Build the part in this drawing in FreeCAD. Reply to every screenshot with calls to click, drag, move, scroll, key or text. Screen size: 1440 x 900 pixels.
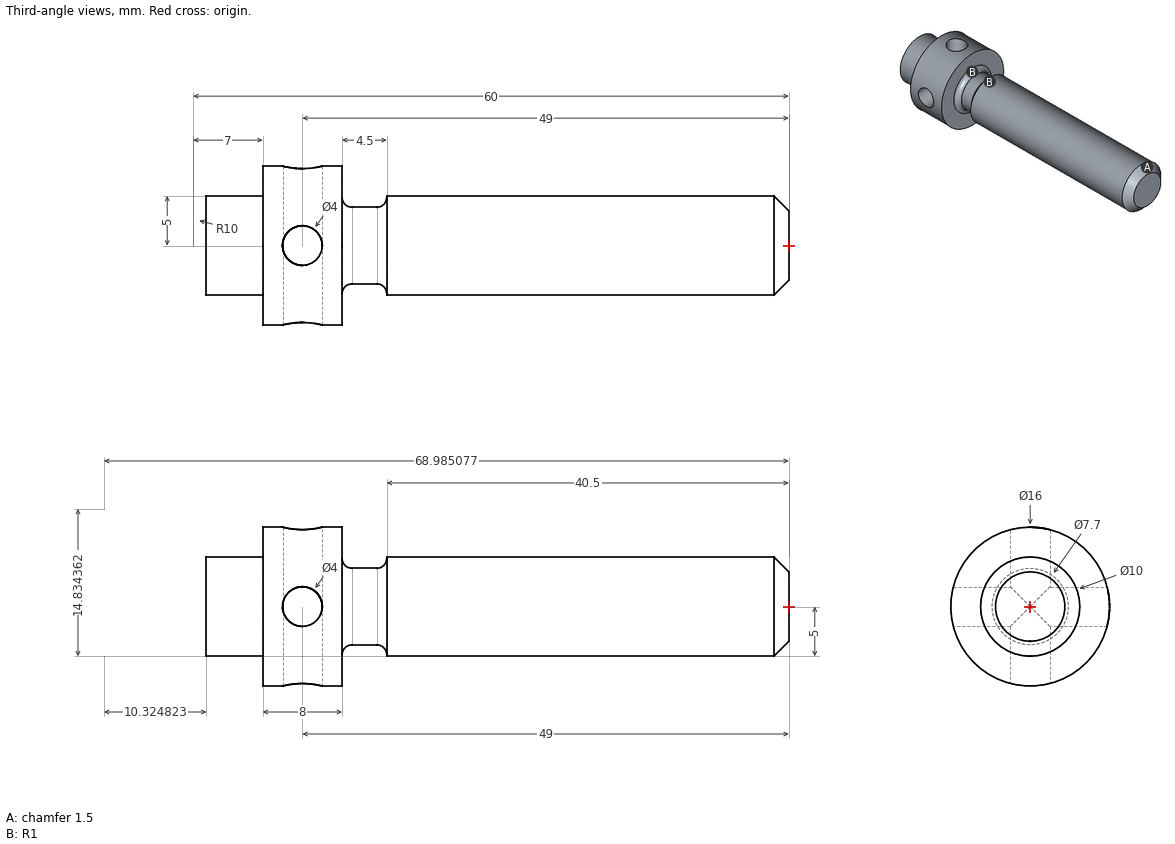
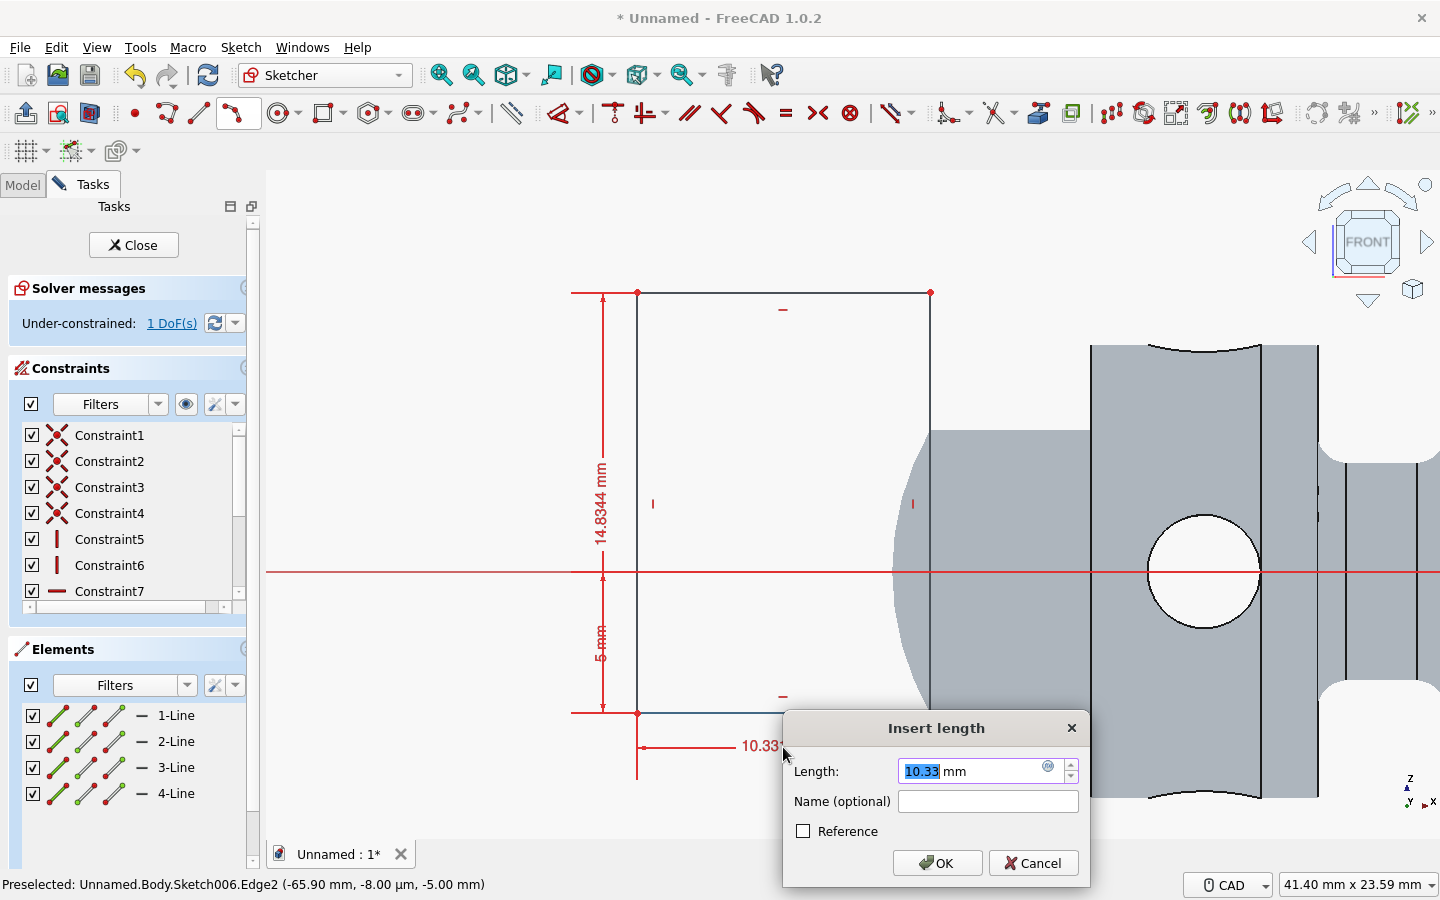
text(10.324823)
key(Return)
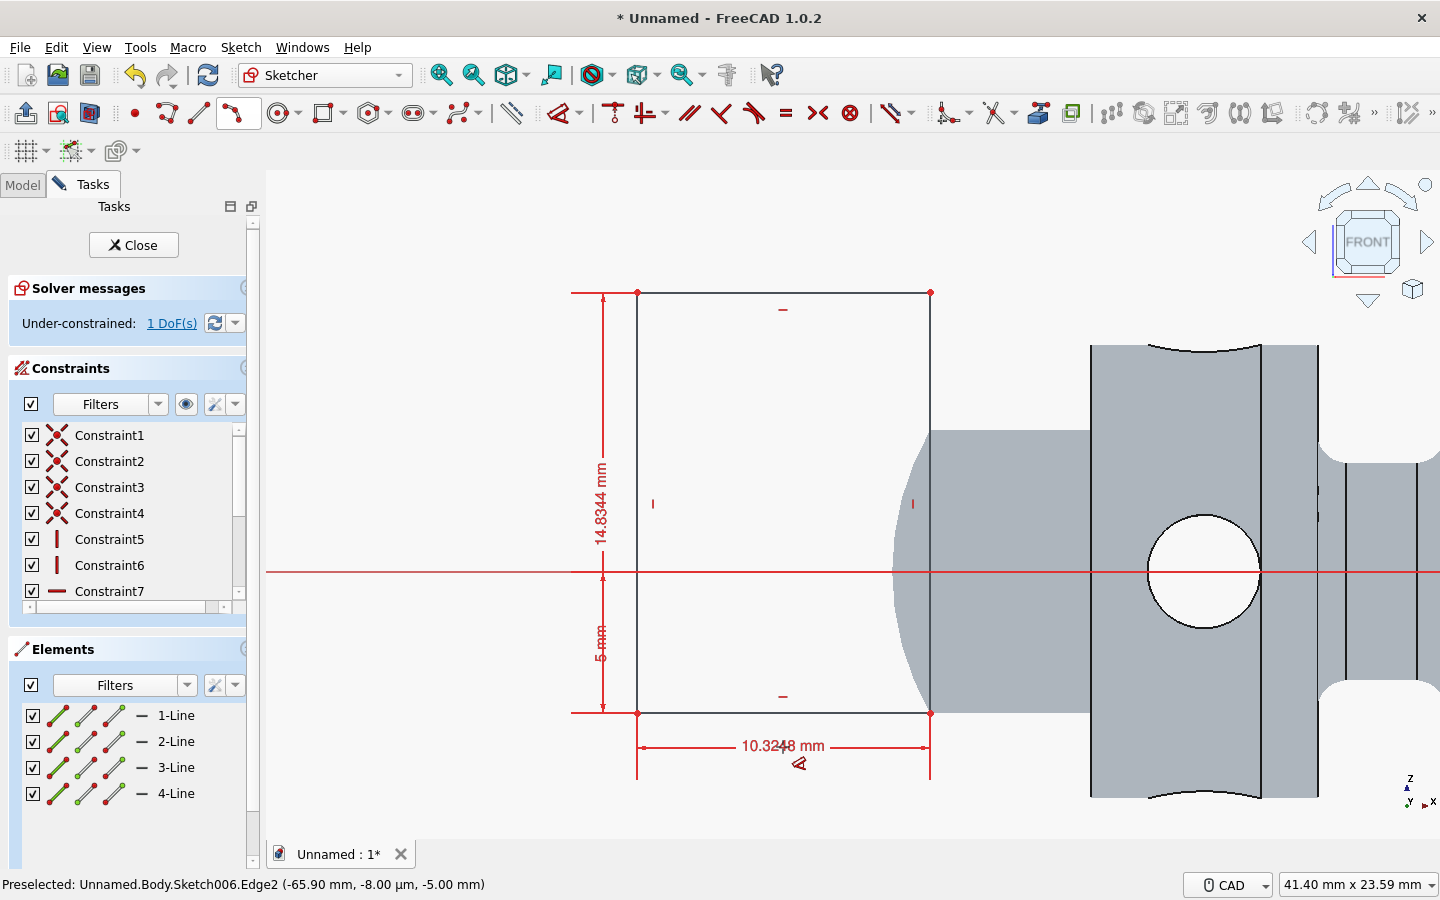
click(637, 293)
click(956, 259)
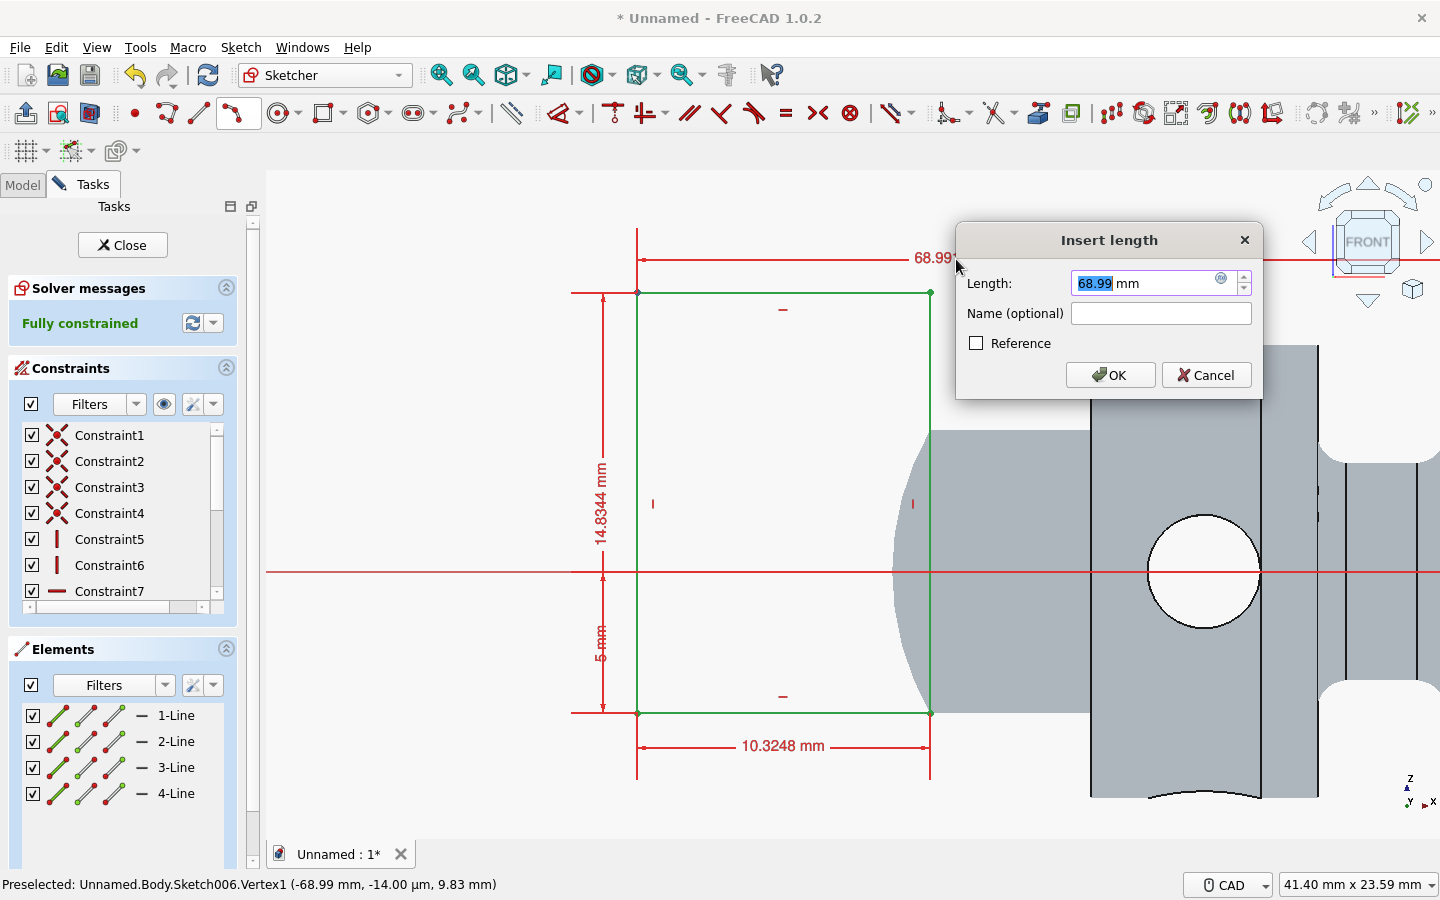
text(68.985077)
key(Return)
key(Escape)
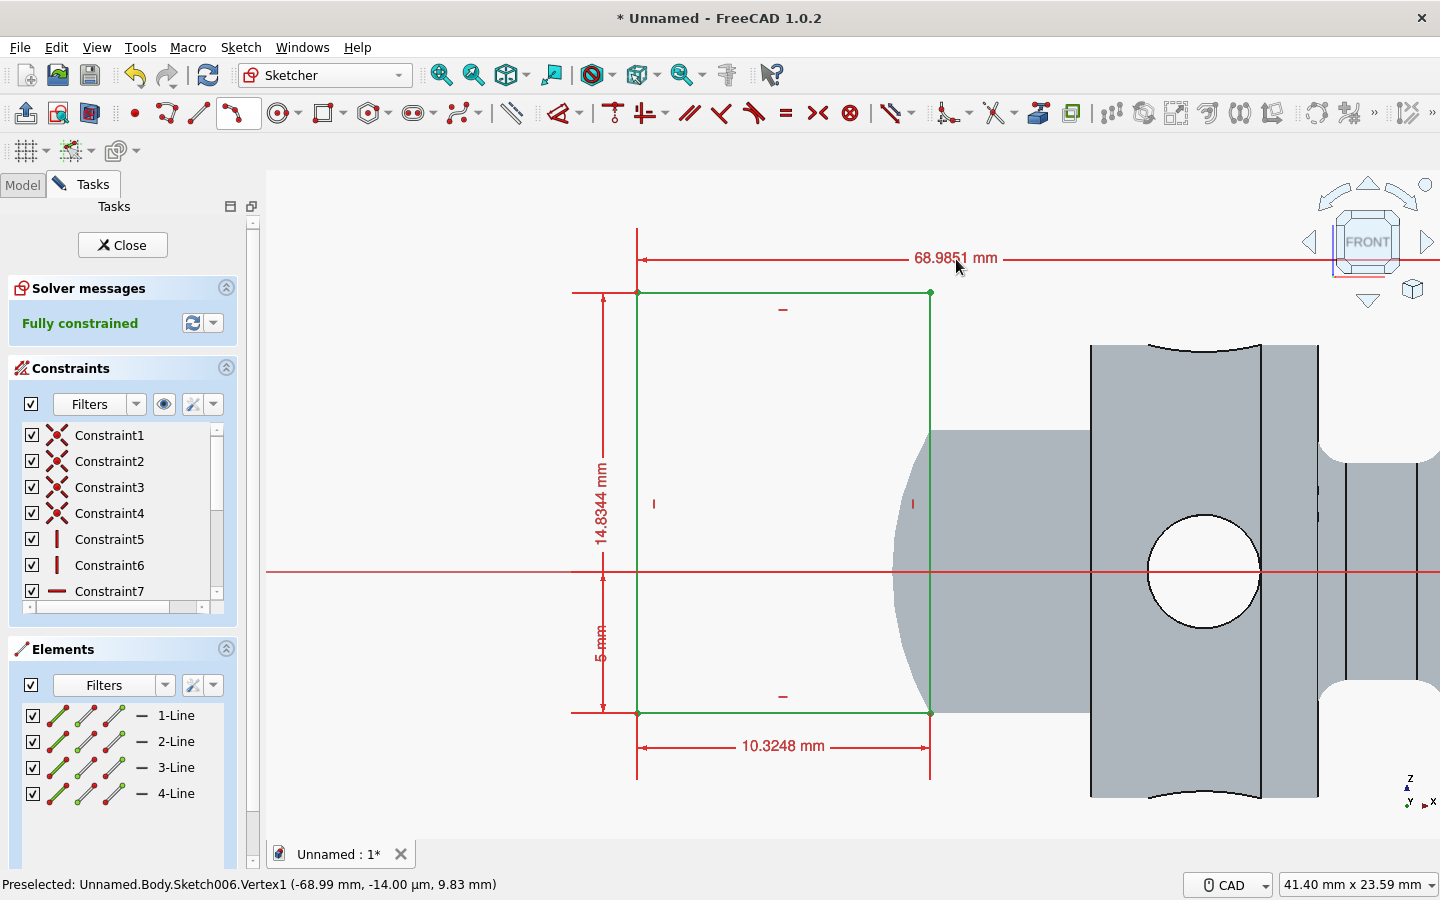
click(123, 245)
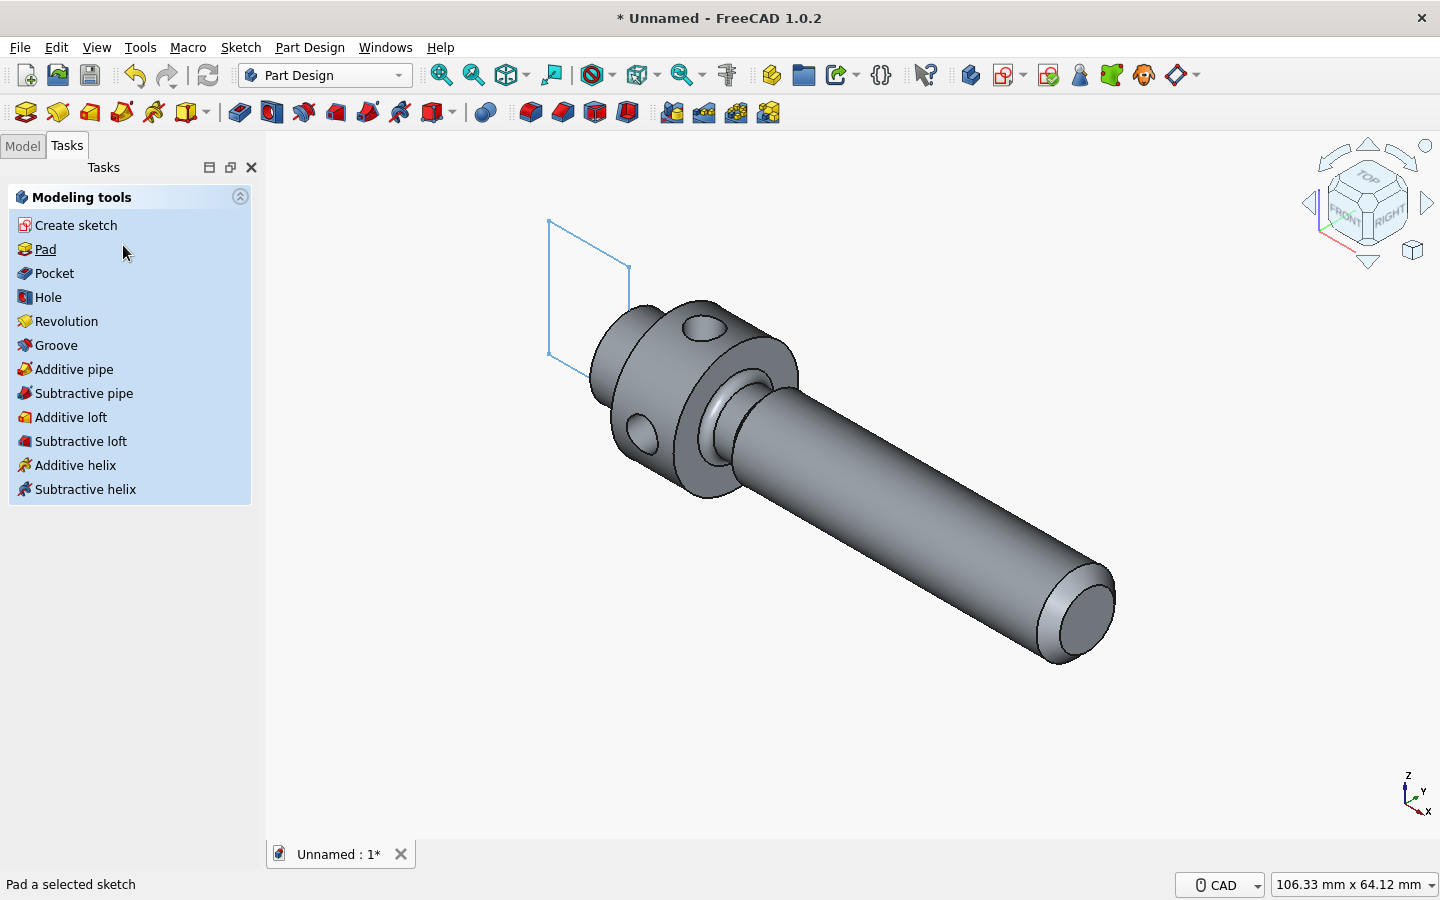
click(240, 112)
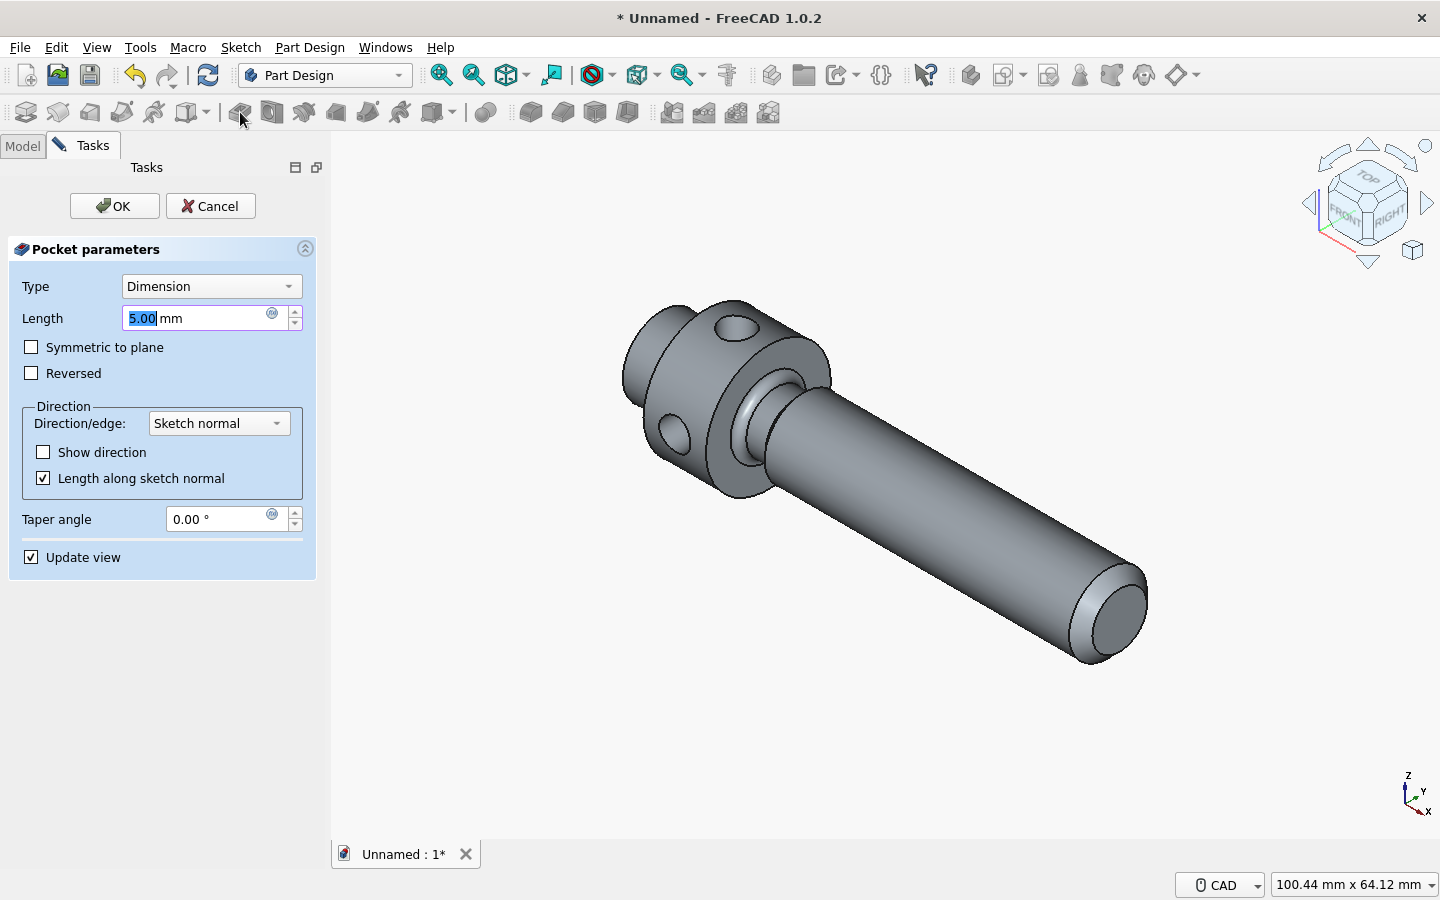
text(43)
key(Tab)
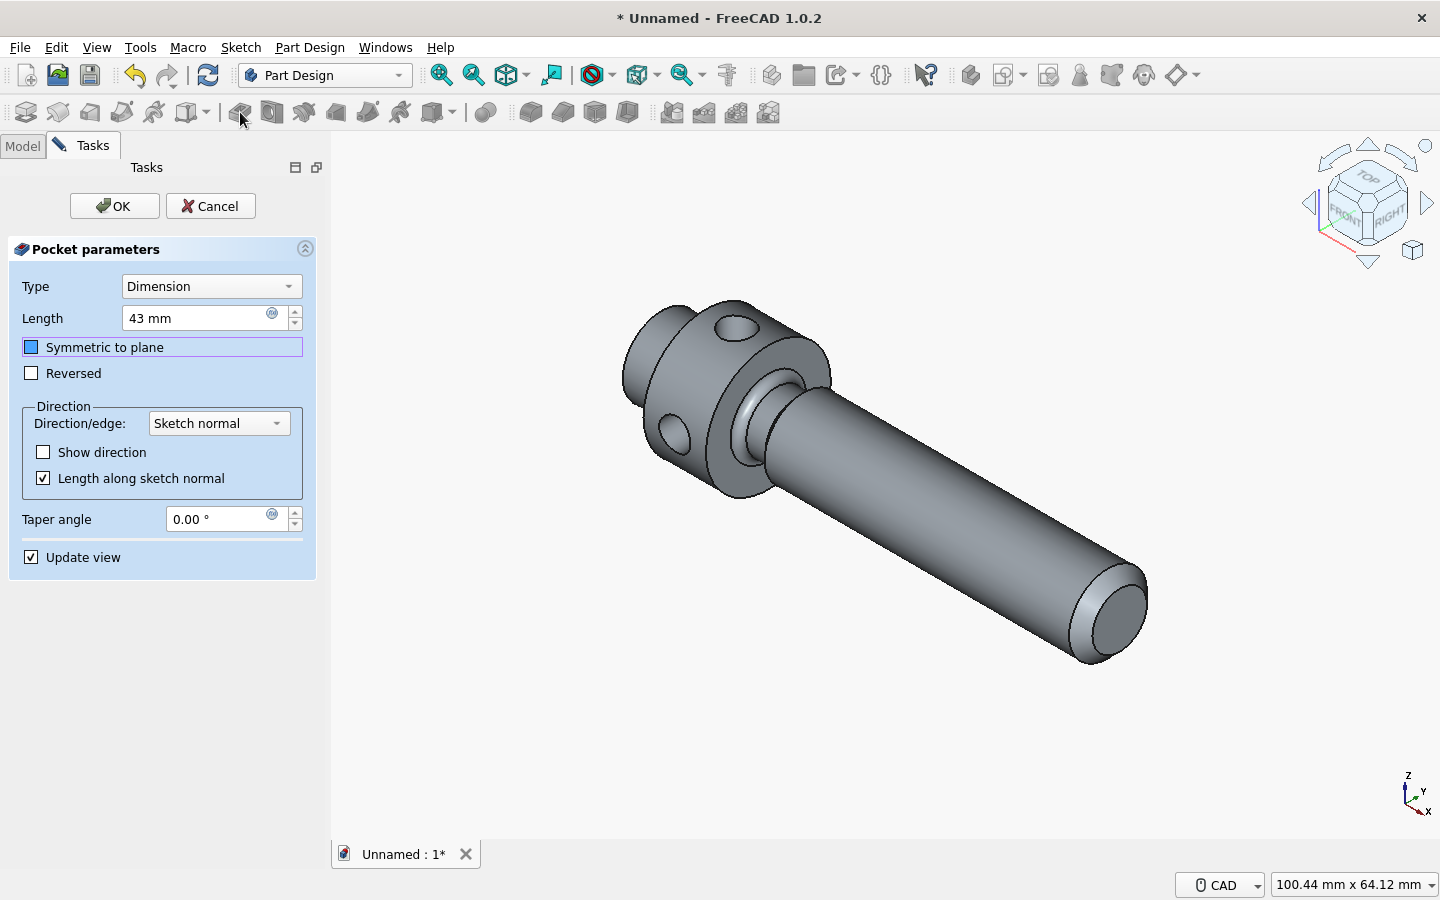
click(30, 347)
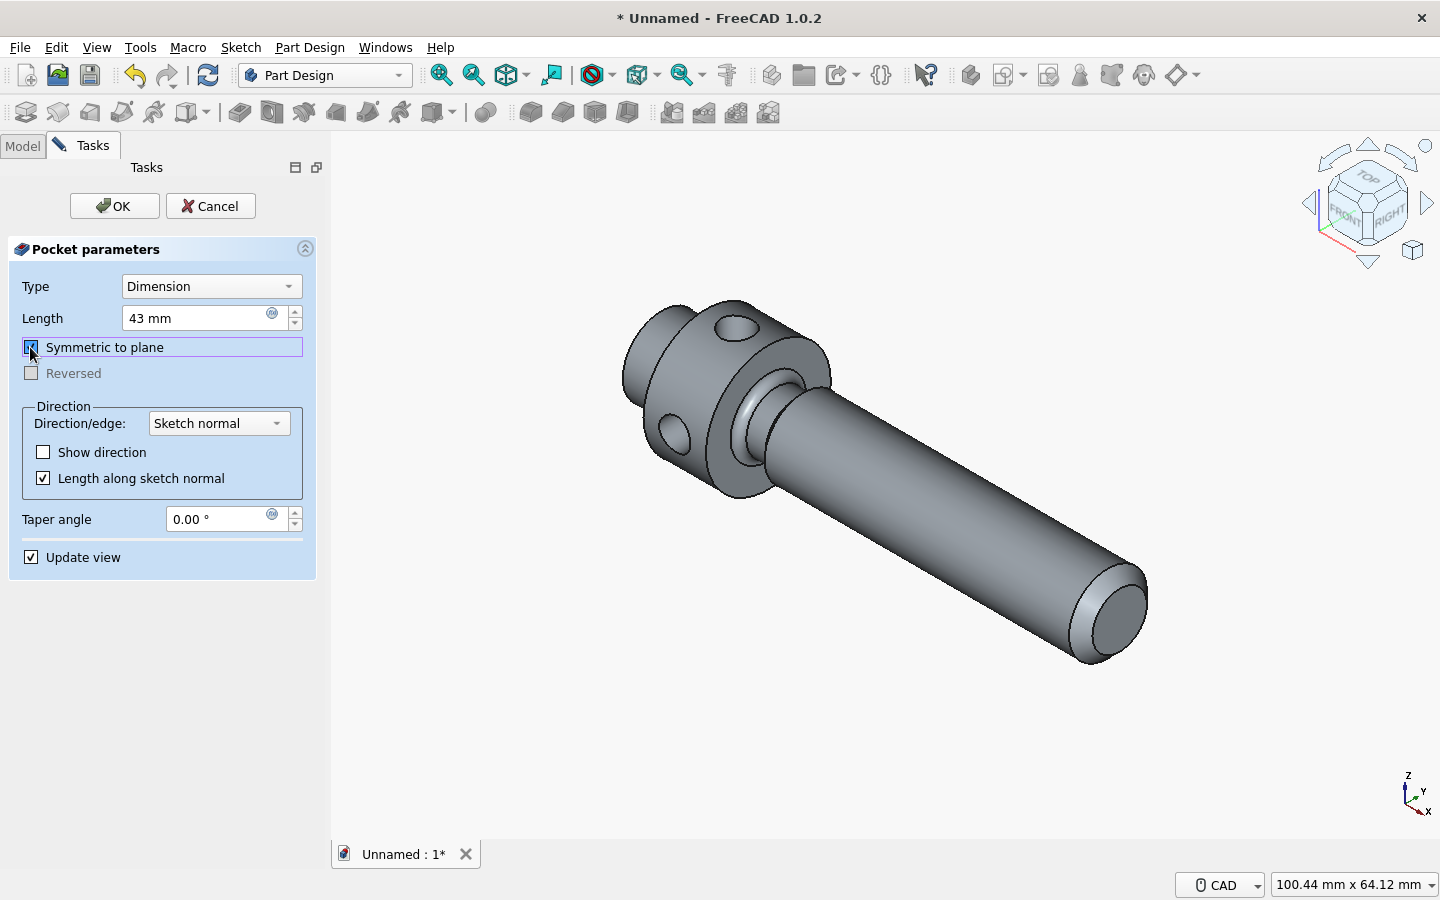
click(115, 206)